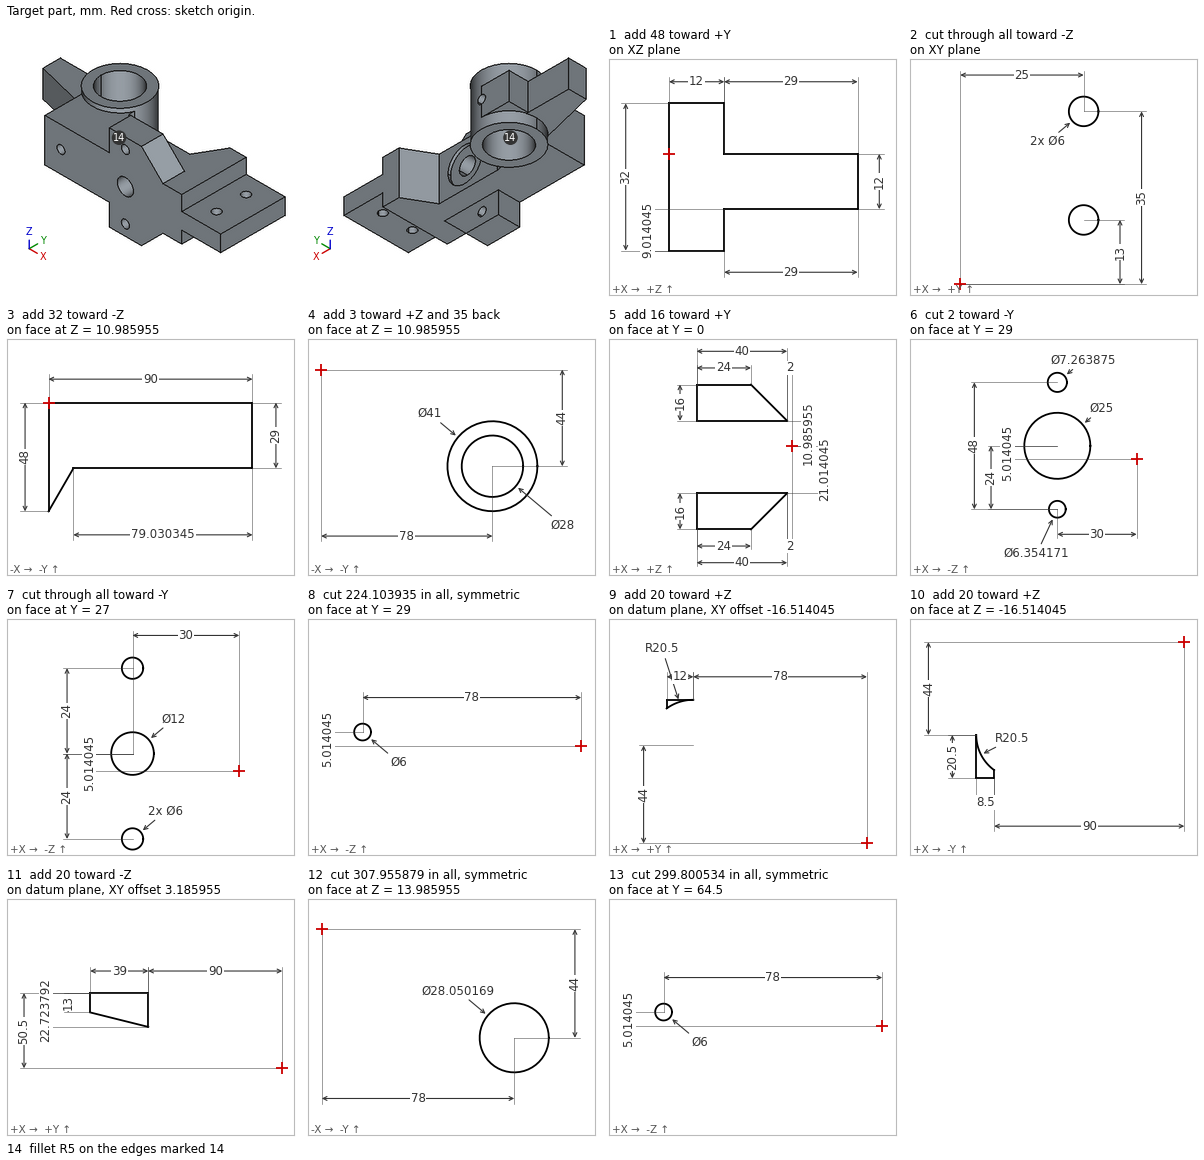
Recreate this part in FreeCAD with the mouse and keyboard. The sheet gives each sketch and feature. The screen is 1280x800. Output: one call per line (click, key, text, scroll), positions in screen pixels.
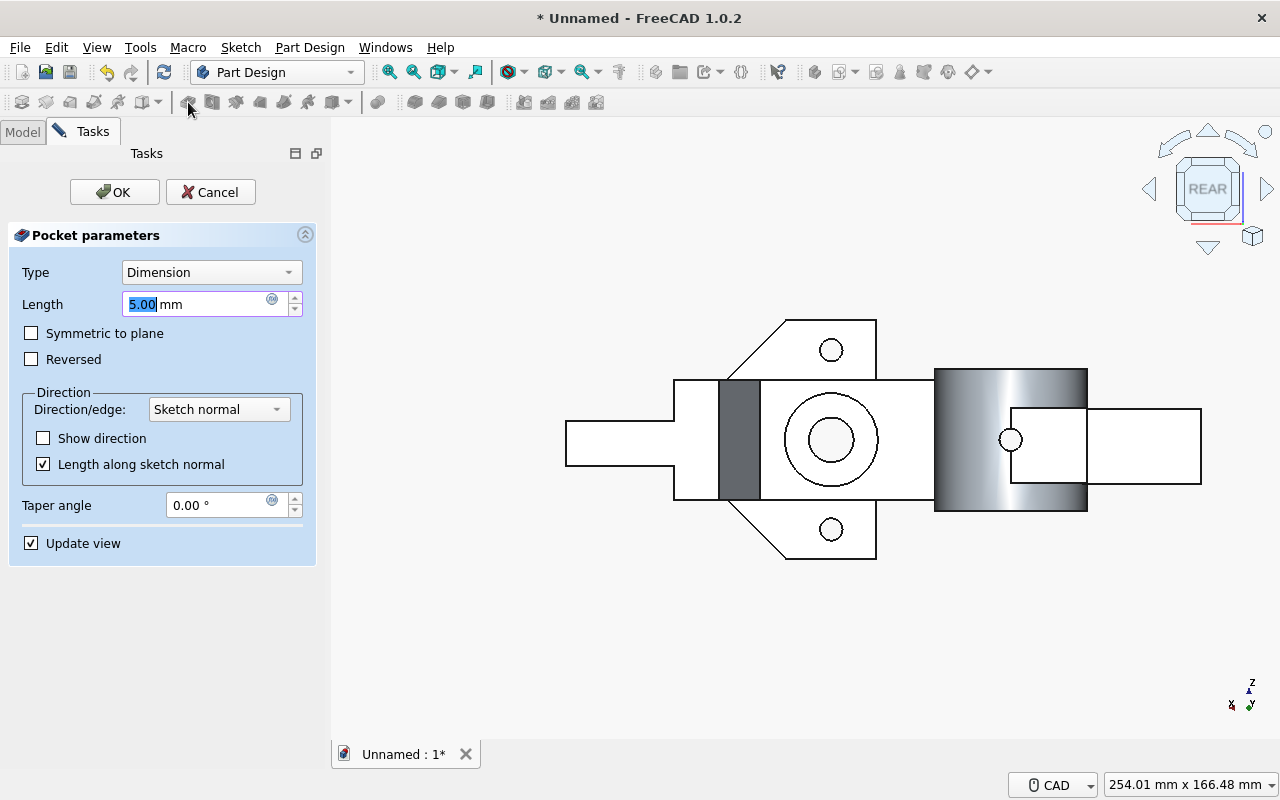
text(299.800534)
key(Tab)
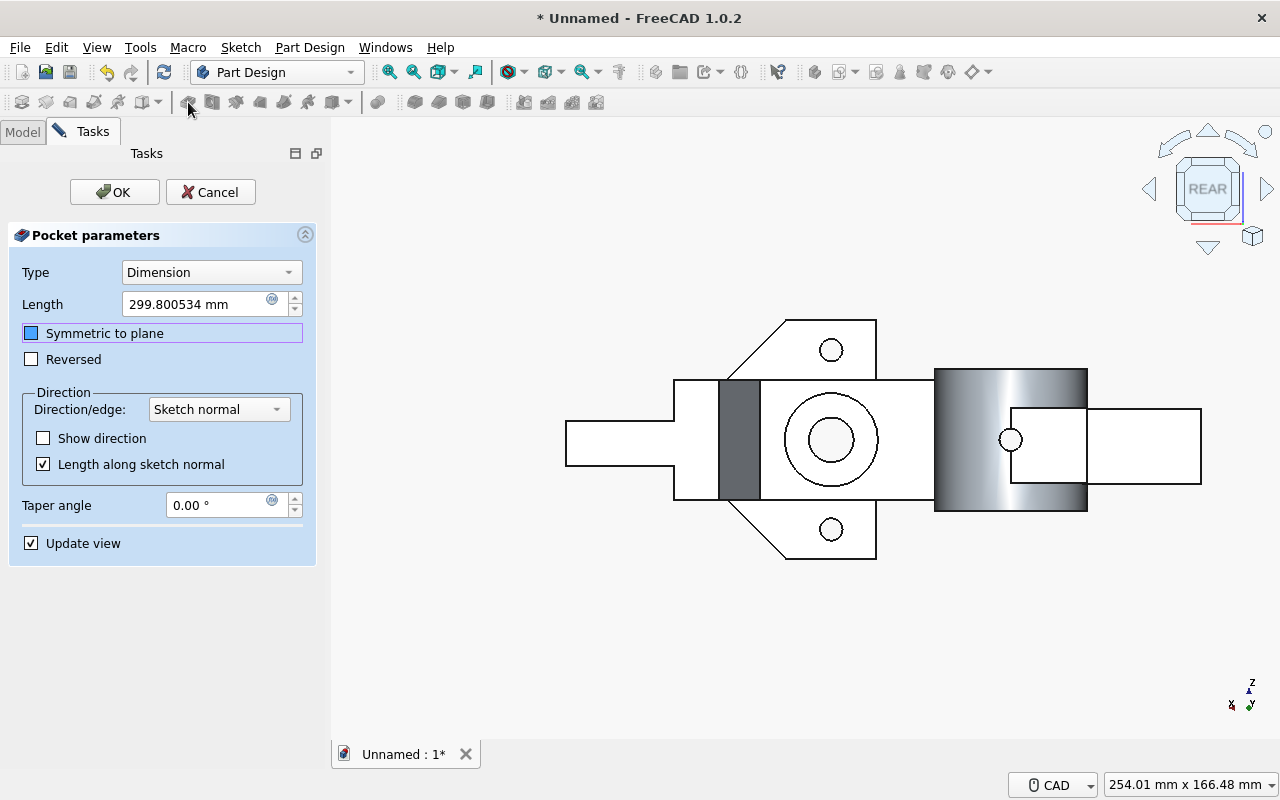
click(30, 333)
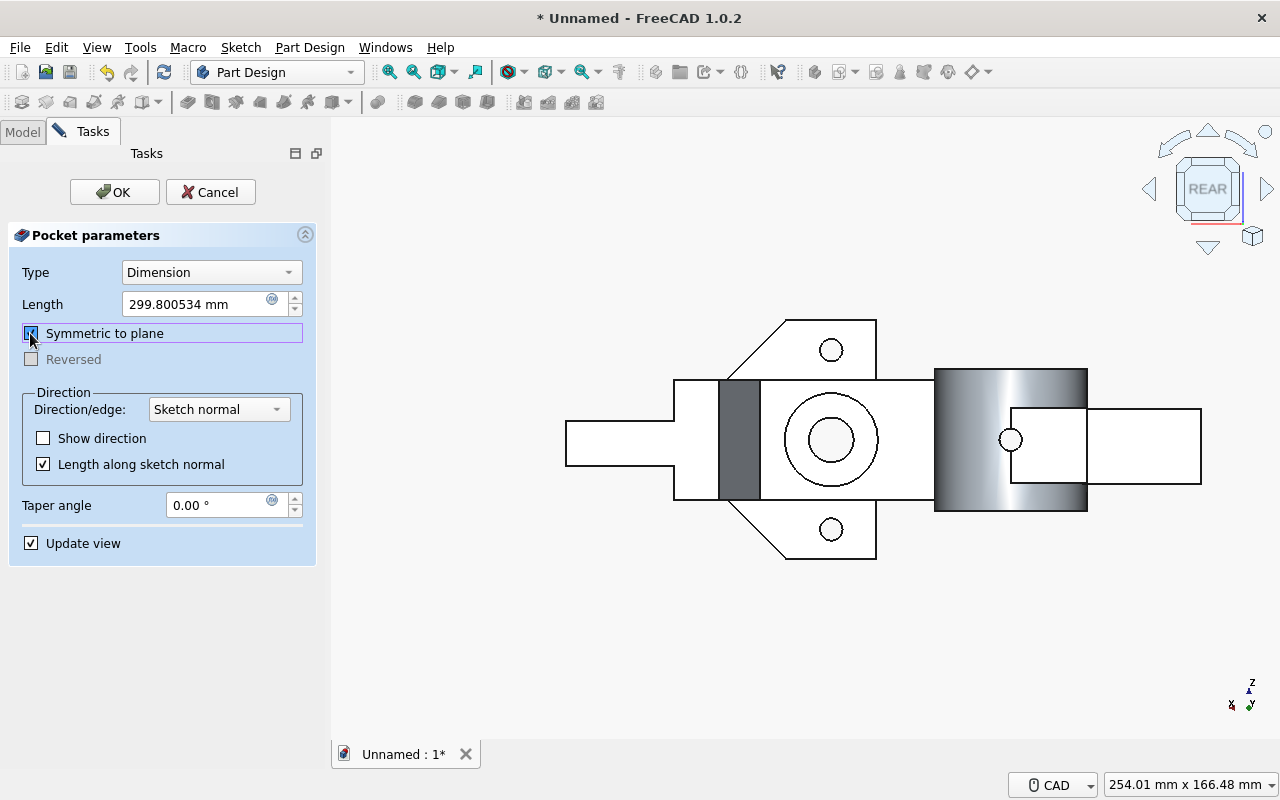
click(115, 192)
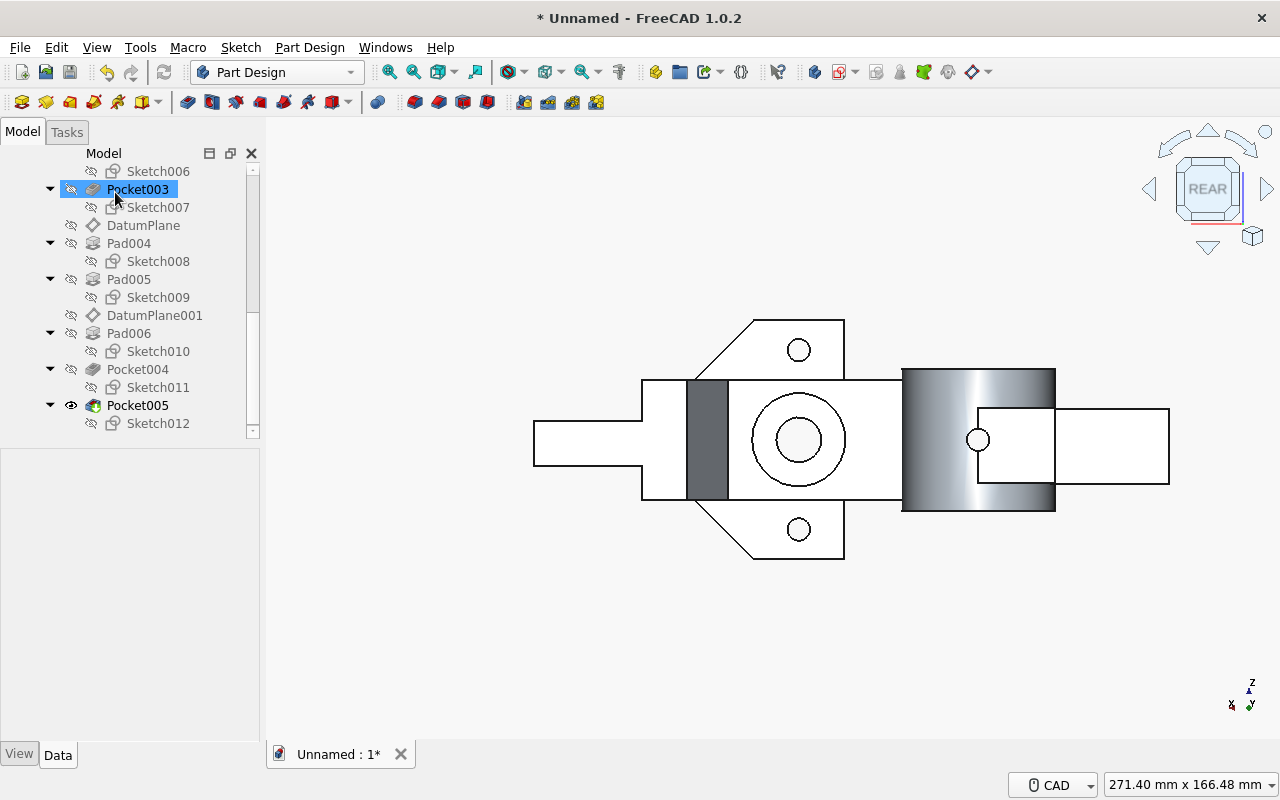
key(0)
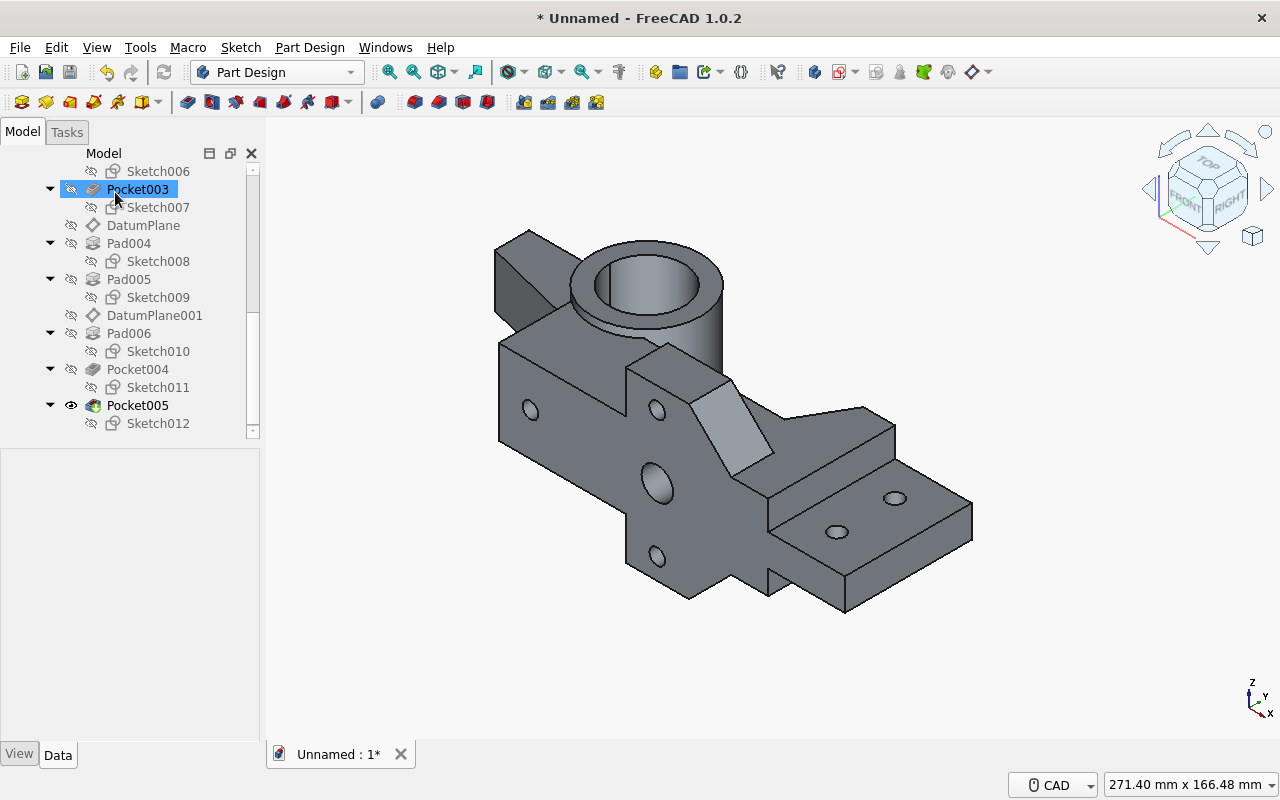
key(2)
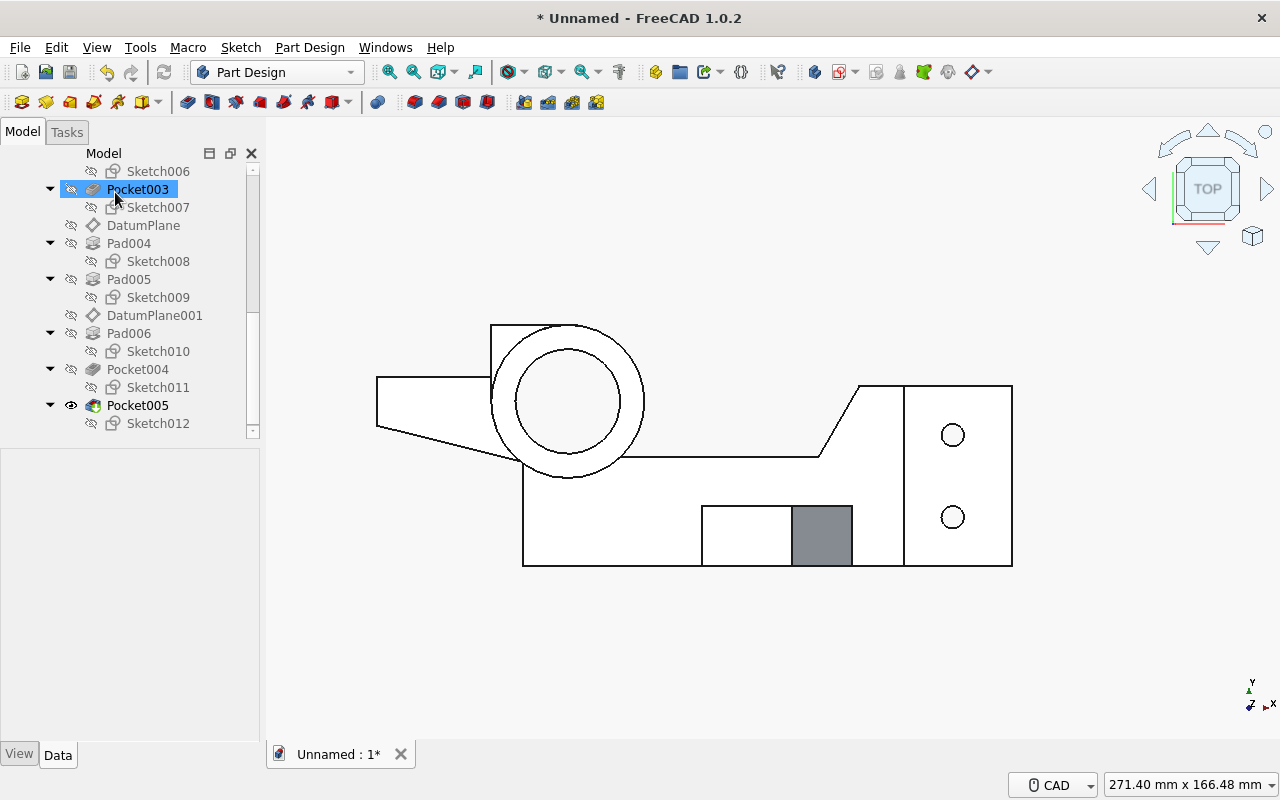
key(1)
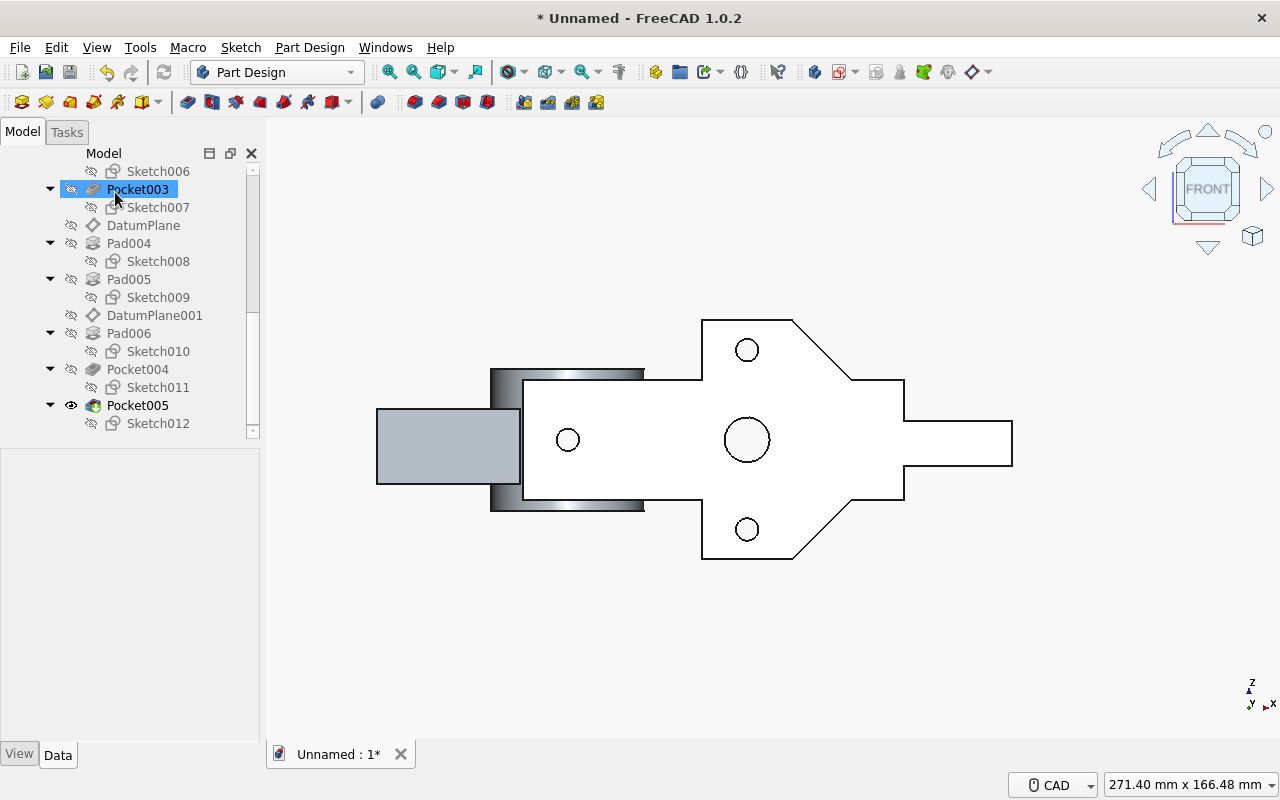
key(3)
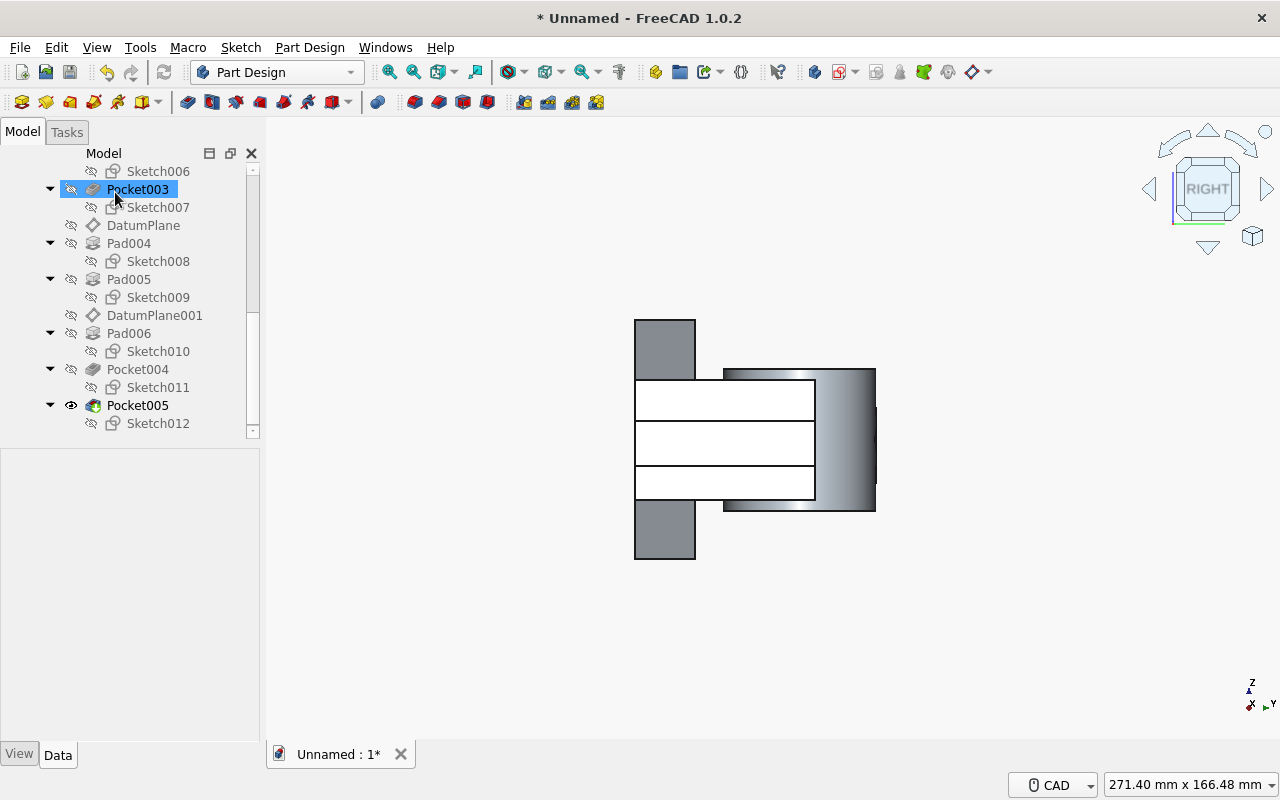
key(v)
key(f)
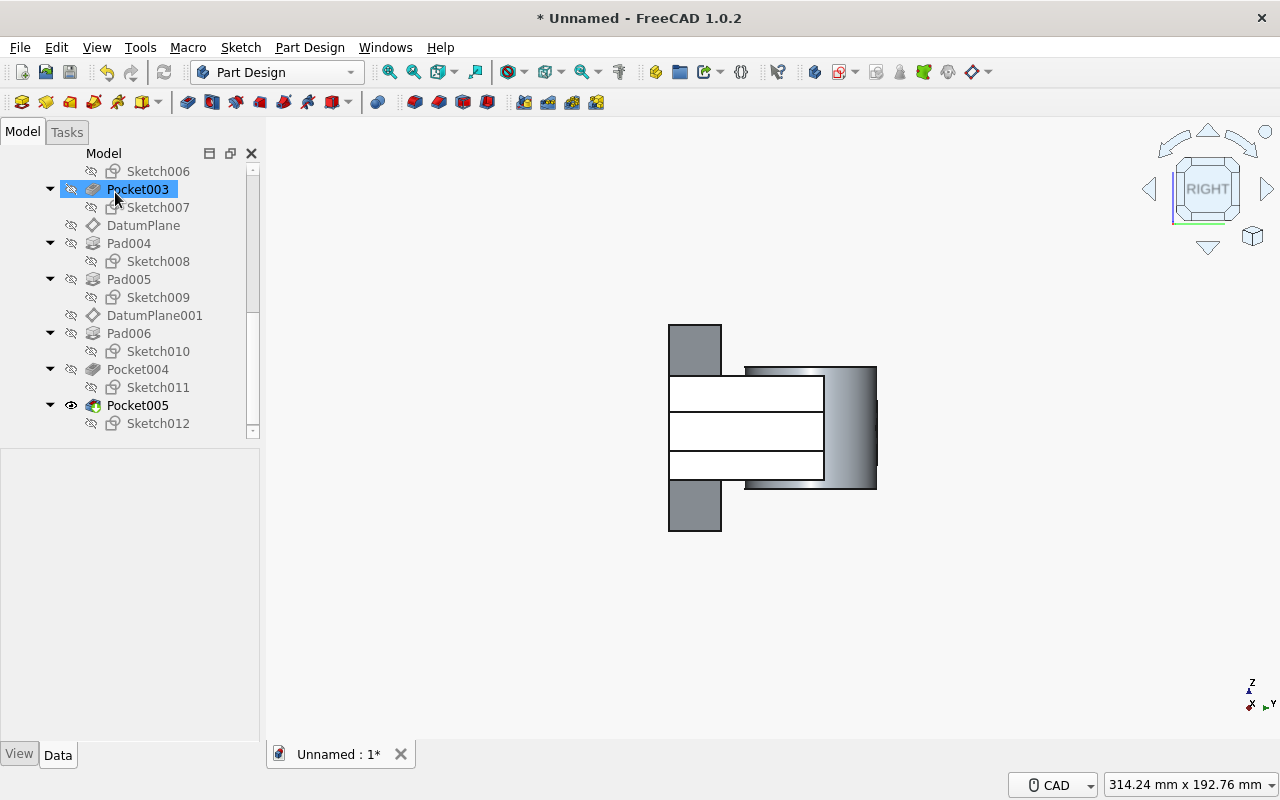
key(5)